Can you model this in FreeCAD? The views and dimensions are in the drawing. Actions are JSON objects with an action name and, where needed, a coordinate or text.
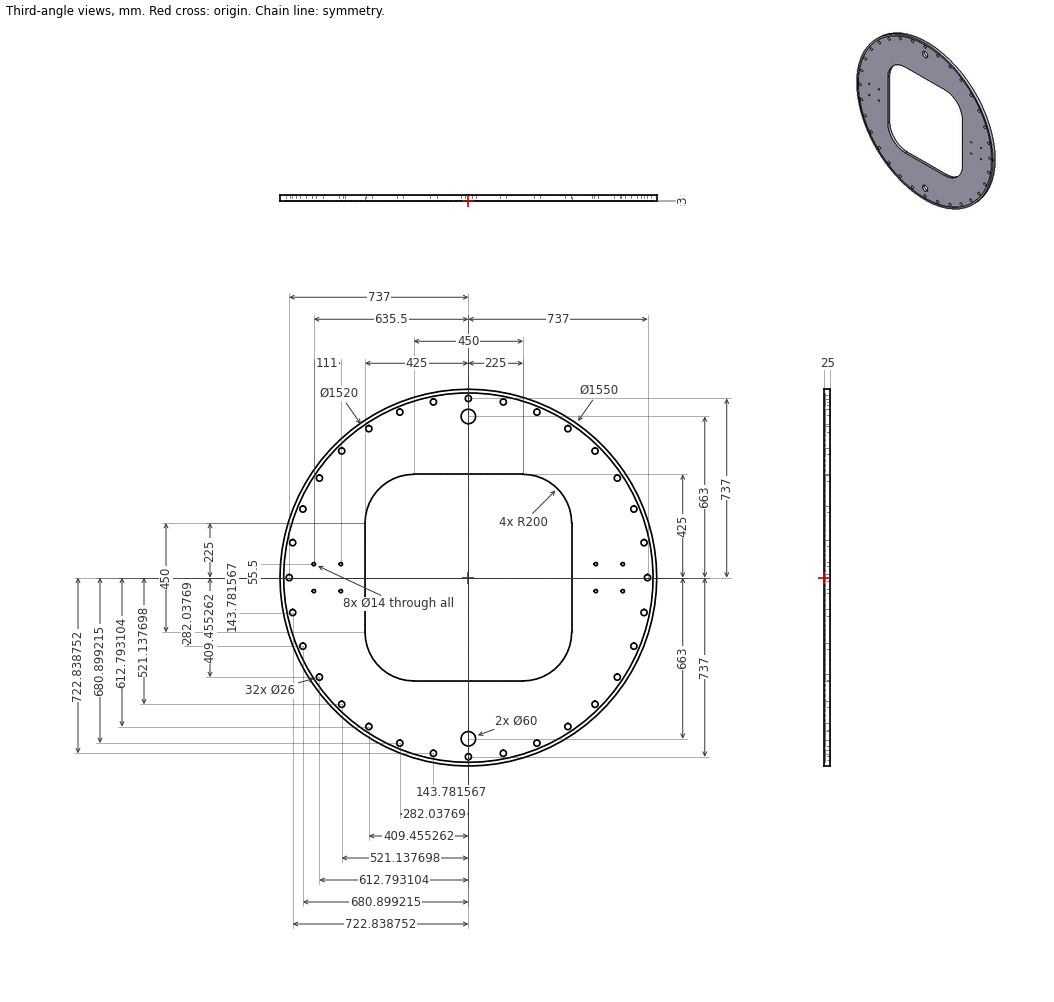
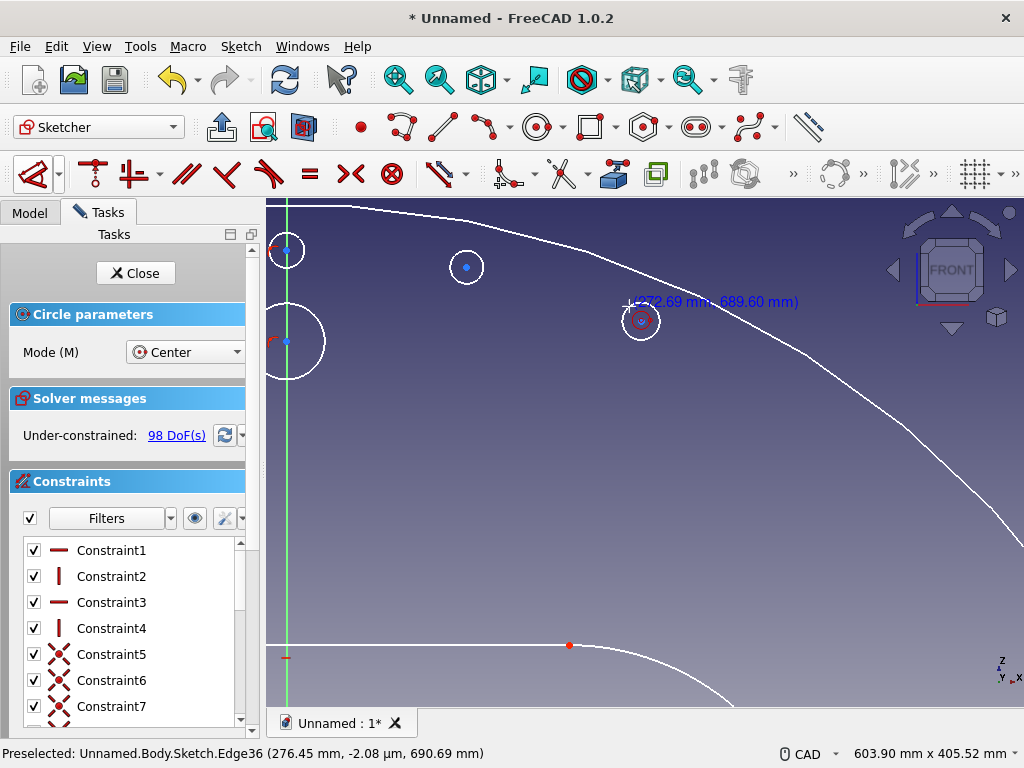
{"action": "scroll", "coordinate": [634, 310], "scroll_direction": "down", "scroll_amount": 9}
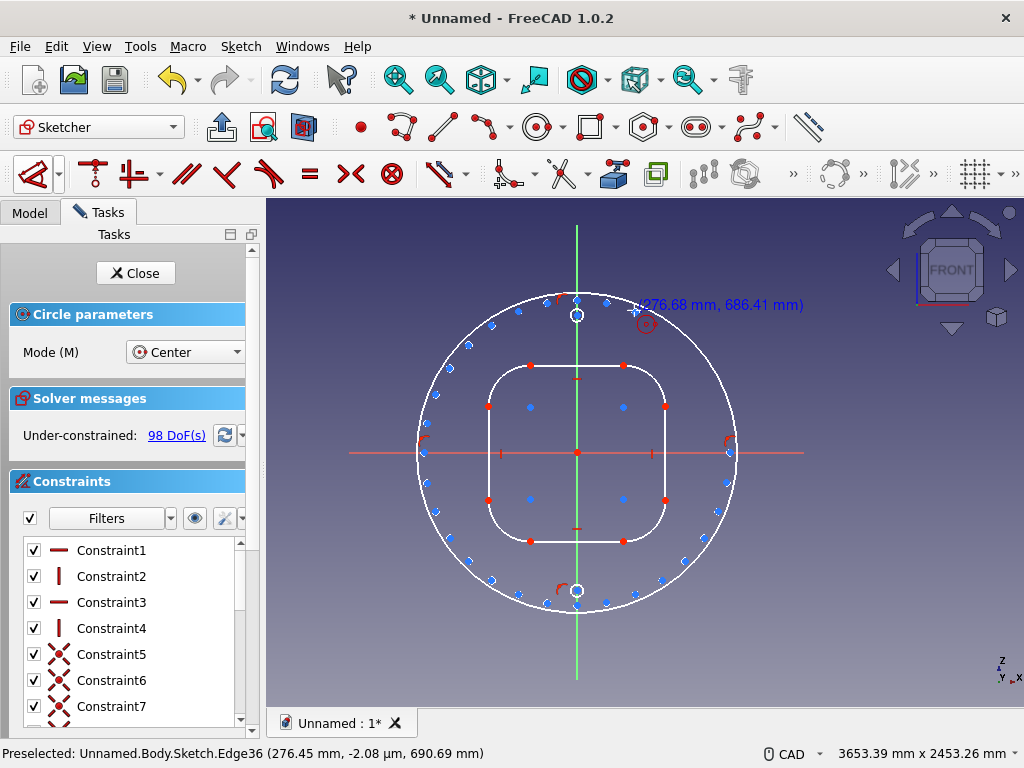
{"action": "scroll", "coordinate": [727, 423], "scroll_direction": "up", "scroll_amount": 11}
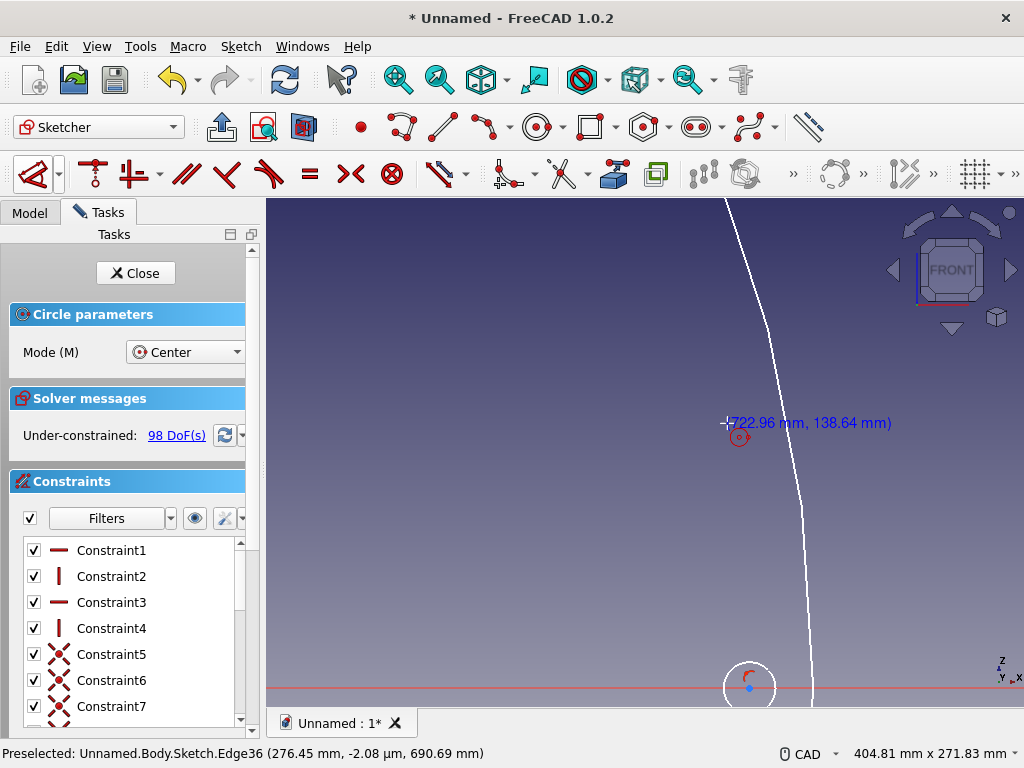
{"action": "scroll", "coordinate": [727, 423], "scroll_direction": "down", "scroll_amount": 11}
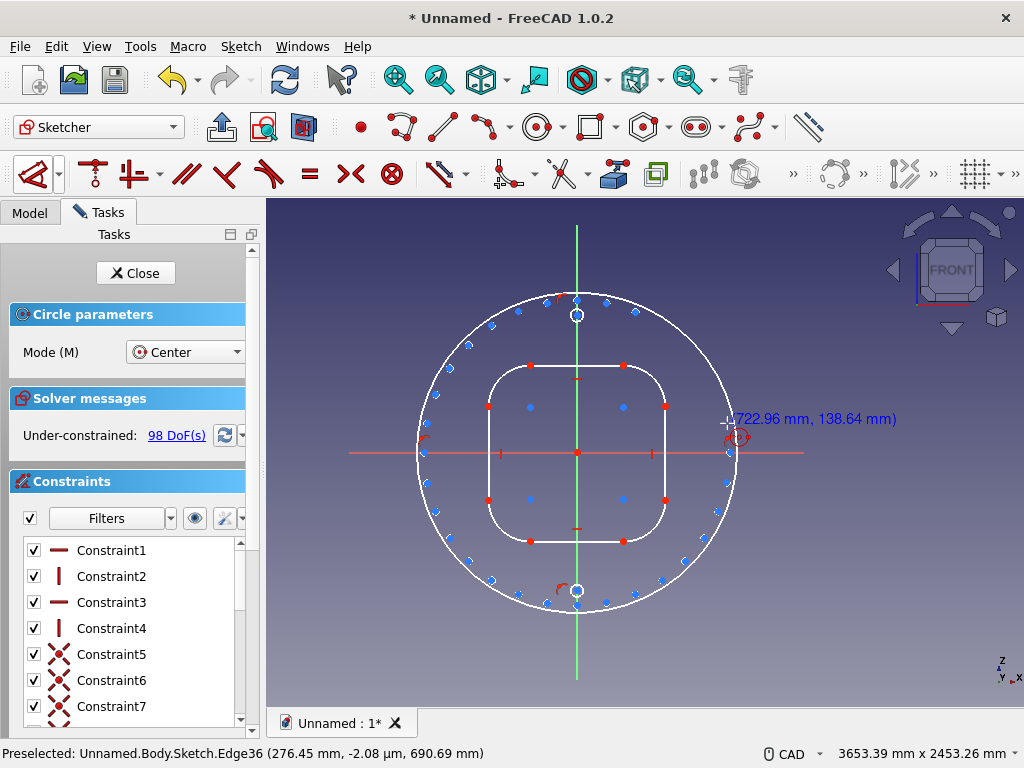
{"action": "scroll", "coordinate": [727, 423], "scroll_direction": "up", "scroll_amount": 4}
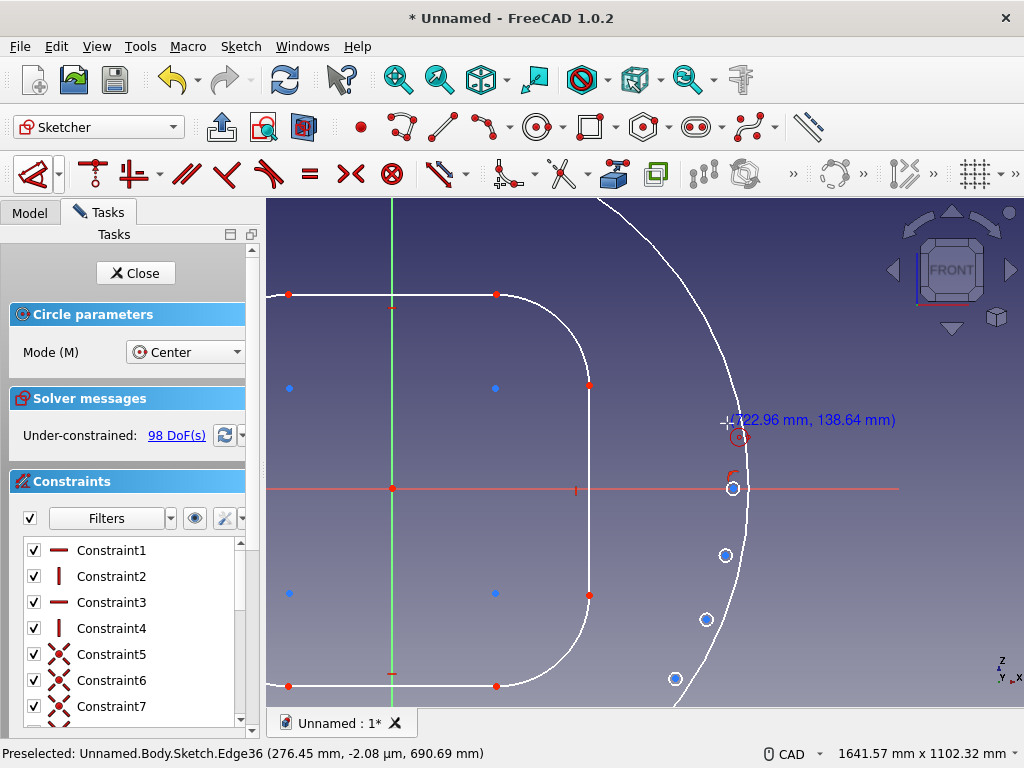
{"action": "left_click", "coordinate": [726, 422]}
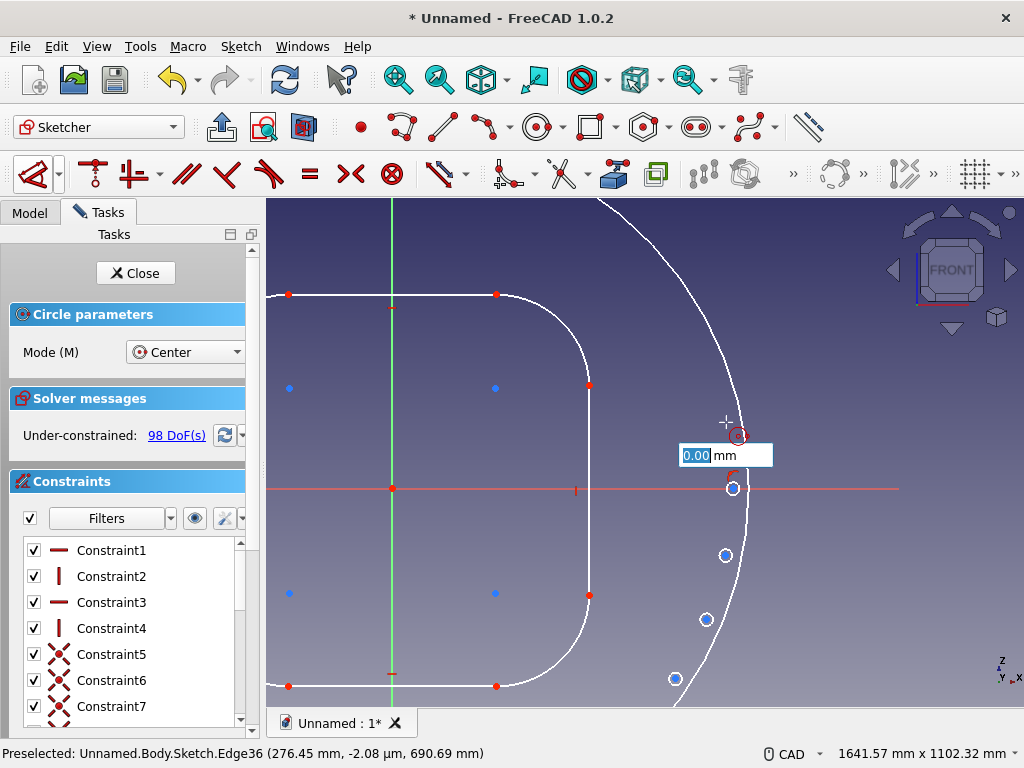
{"action": "scroll", "coordinate": [722, 418], "scroll_direction": "up", "scroll_amount": 5}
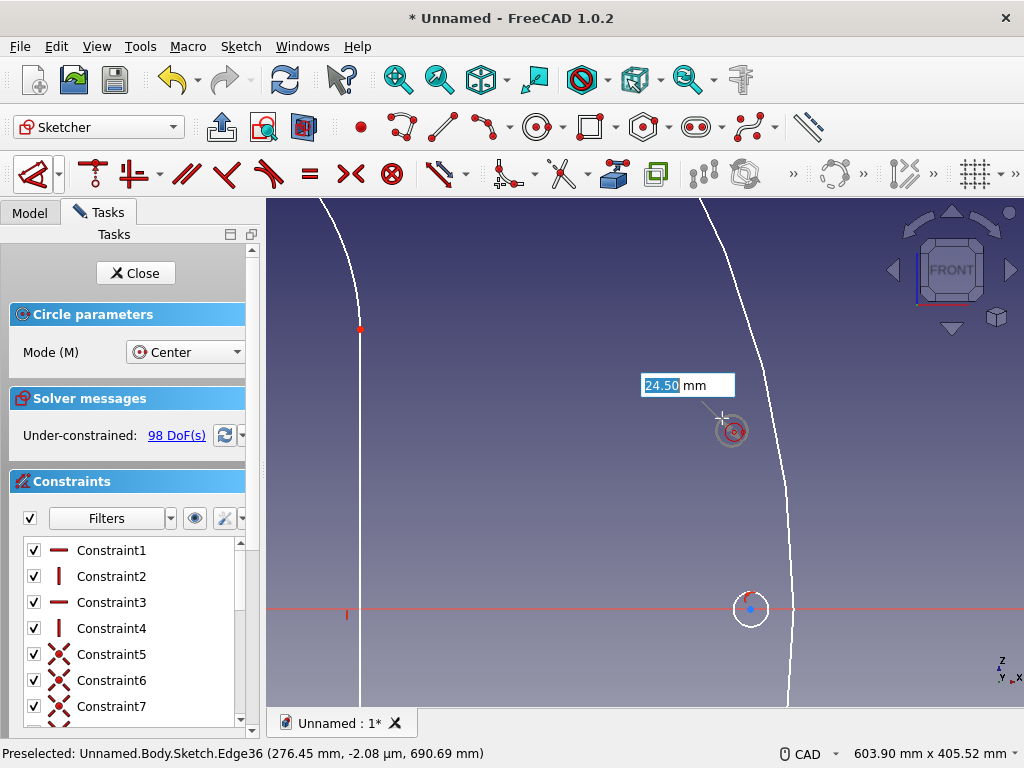
{"action": "left_click", "coordinate": [721, 417]}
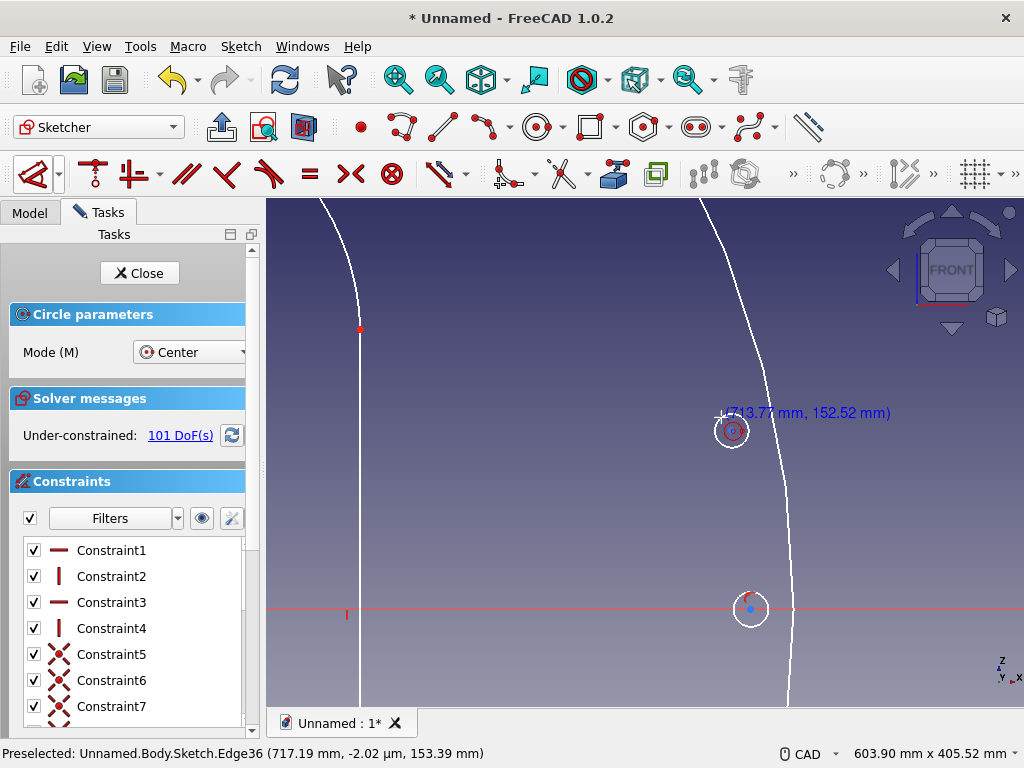
{"action": "scroll", "coordinate": [680, 255], "scroll_direction": "up", "scroll_amount": 2}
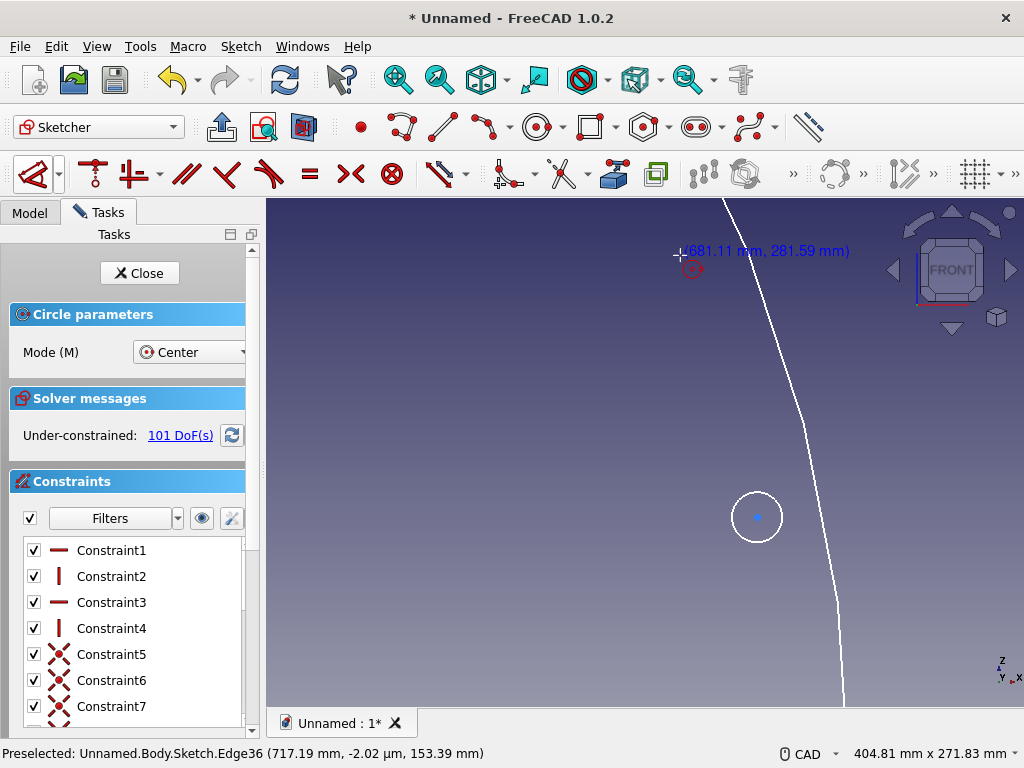
{"action": "scroll", "coordinate": [723, 411], "scroll_direction": "down", "scroll_amount": 11}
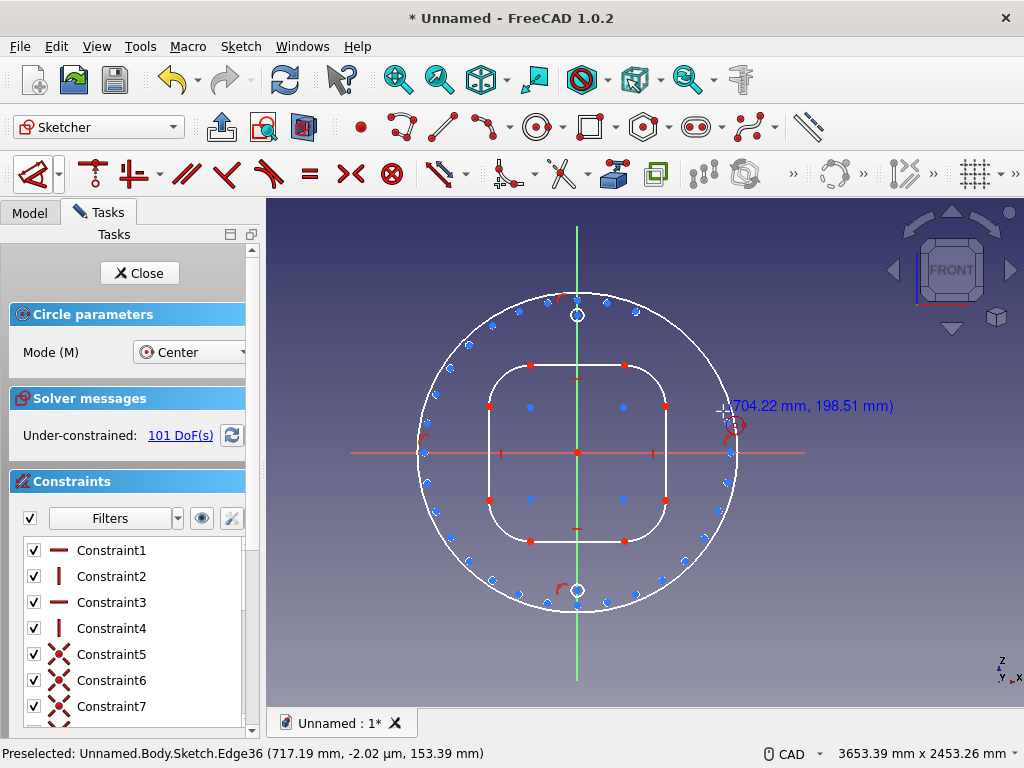
{"action": "scroll", "coordinate": [719, 394], "scroll_direction": "up", "scroll_amount": 4}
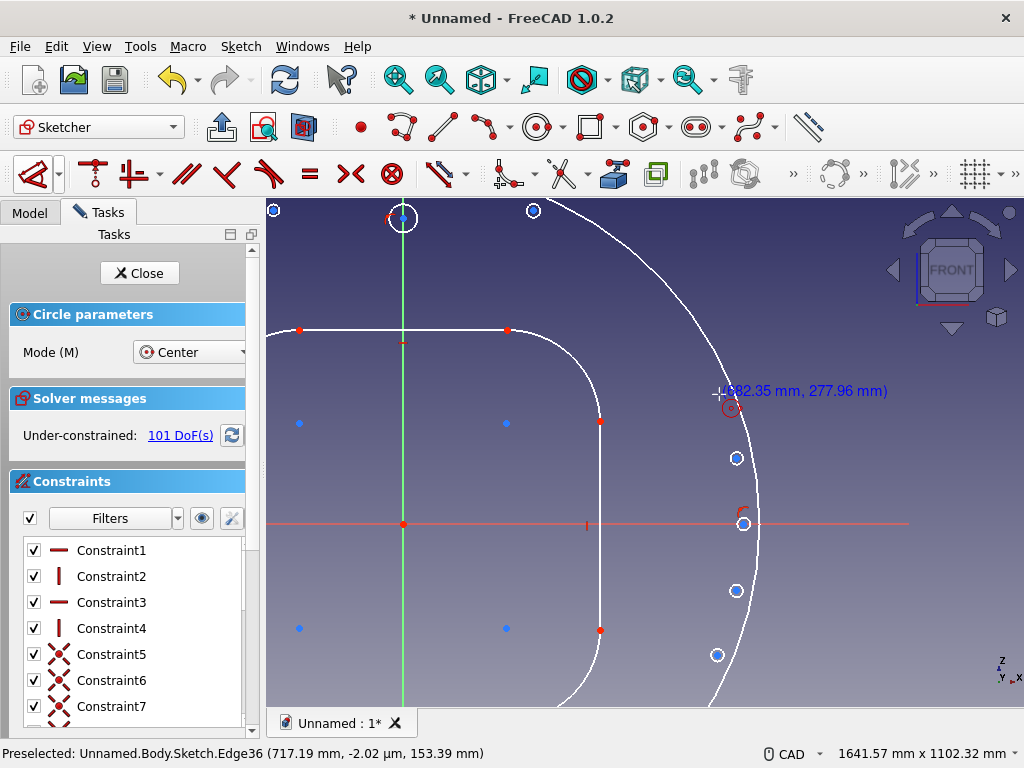
{"action": "left_click", "coordinate": [718, 394]}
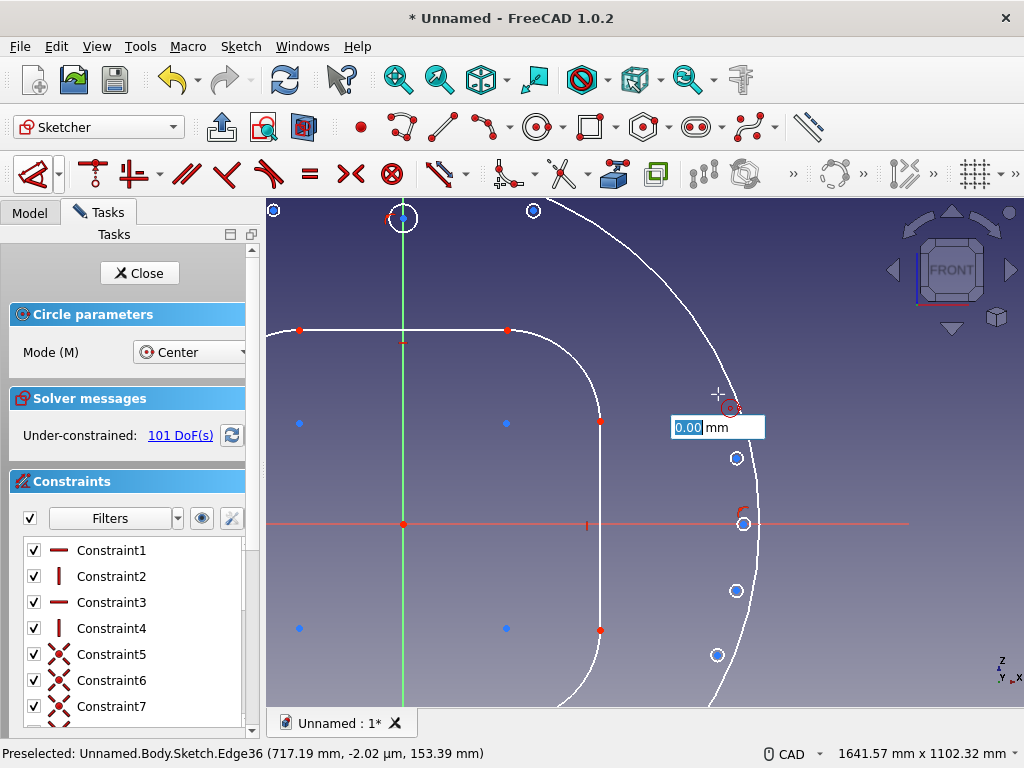
{"action": "scroll", "coordinate": [713, 390], "scroll_direction": "up", "scroll_amount": 5}